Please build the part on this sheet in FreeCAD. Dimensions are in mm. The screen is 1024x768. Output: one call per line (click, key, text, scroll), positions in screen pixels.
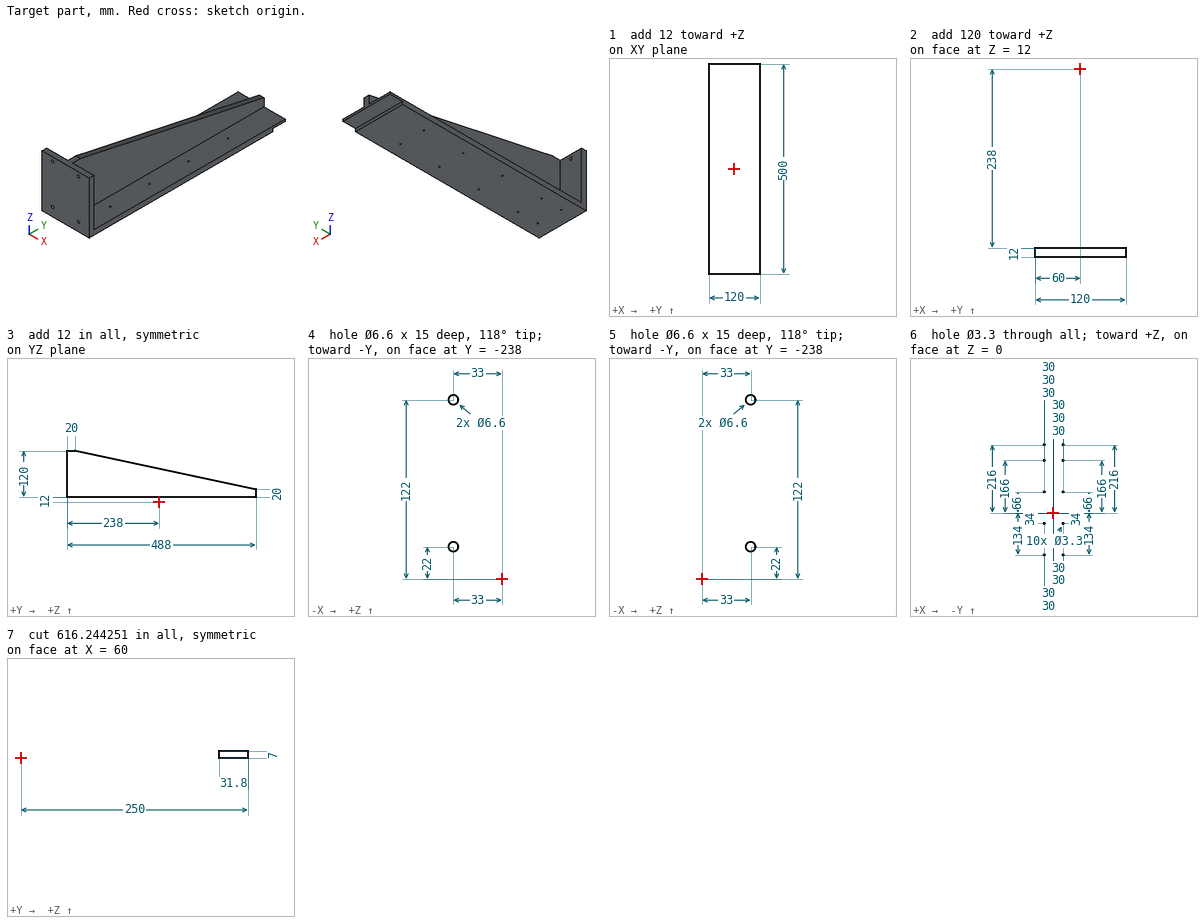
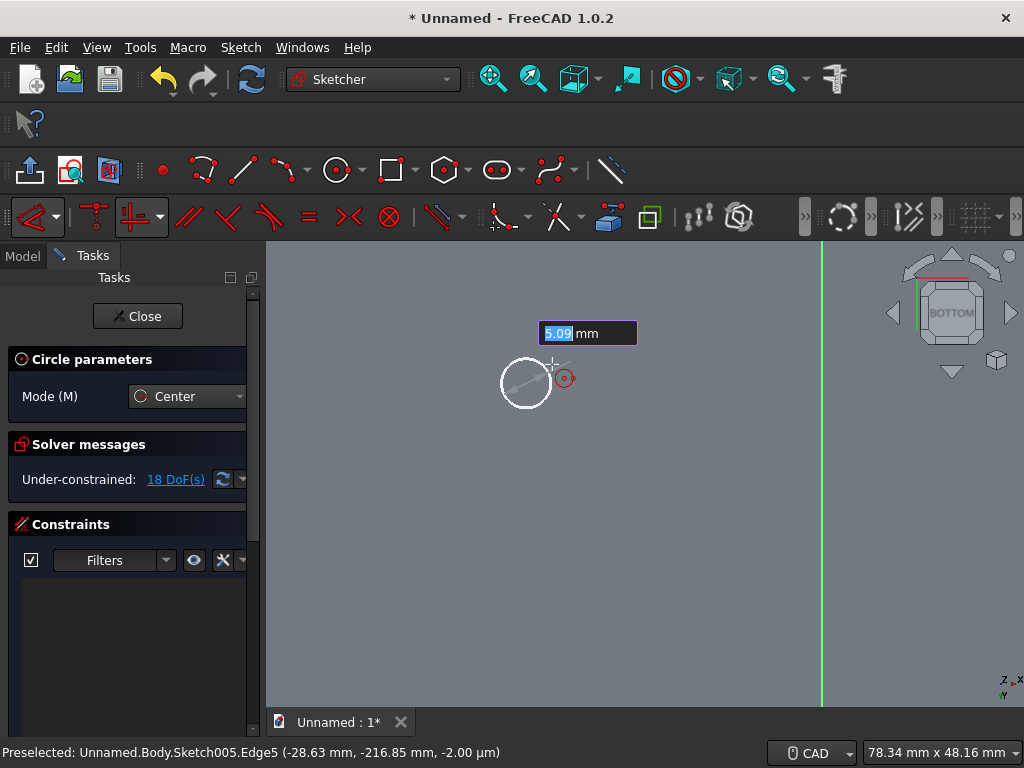
click(543, 356)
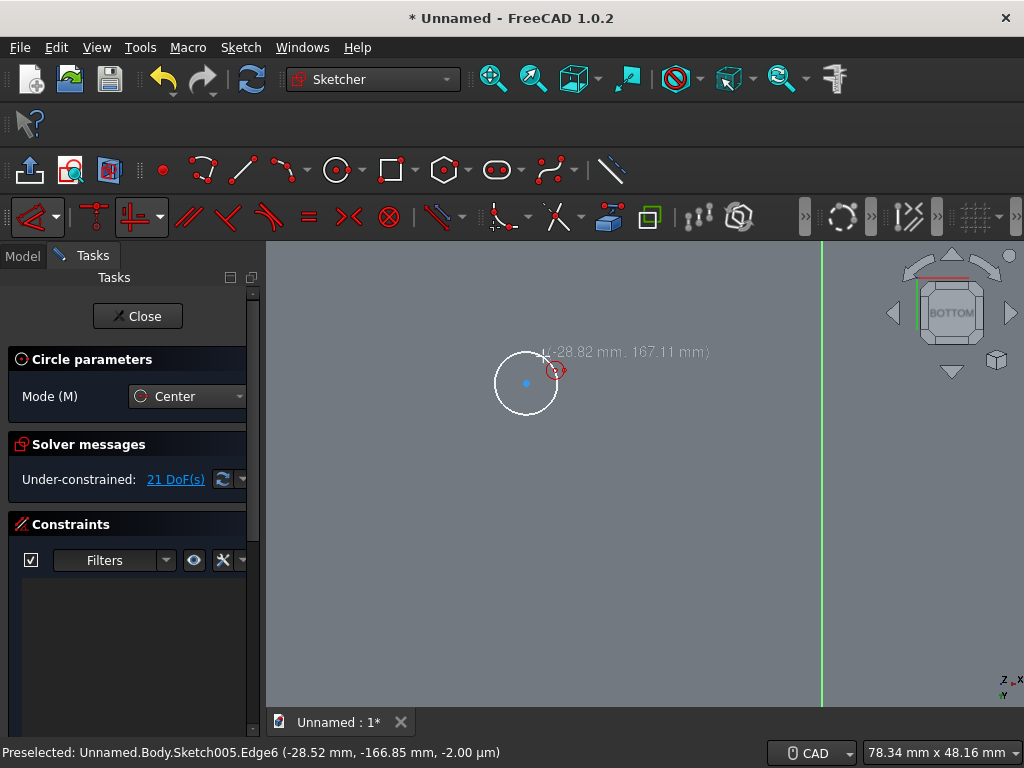
scroll(552, 364, down, 12)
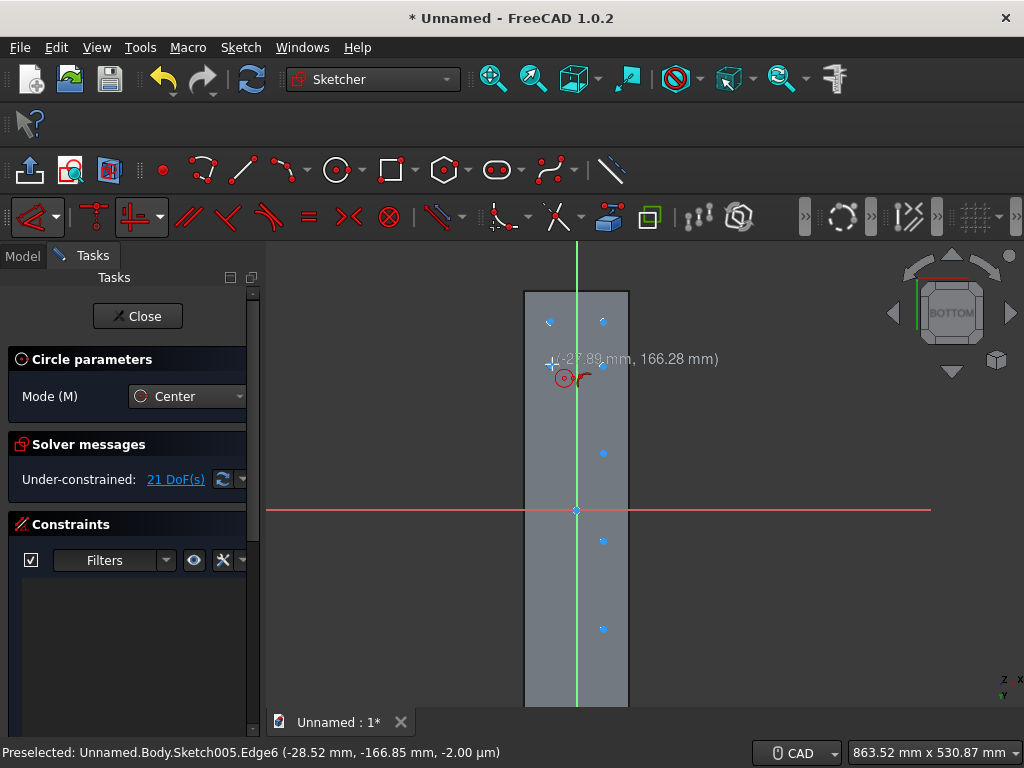
scroll(550, 452, up, 14)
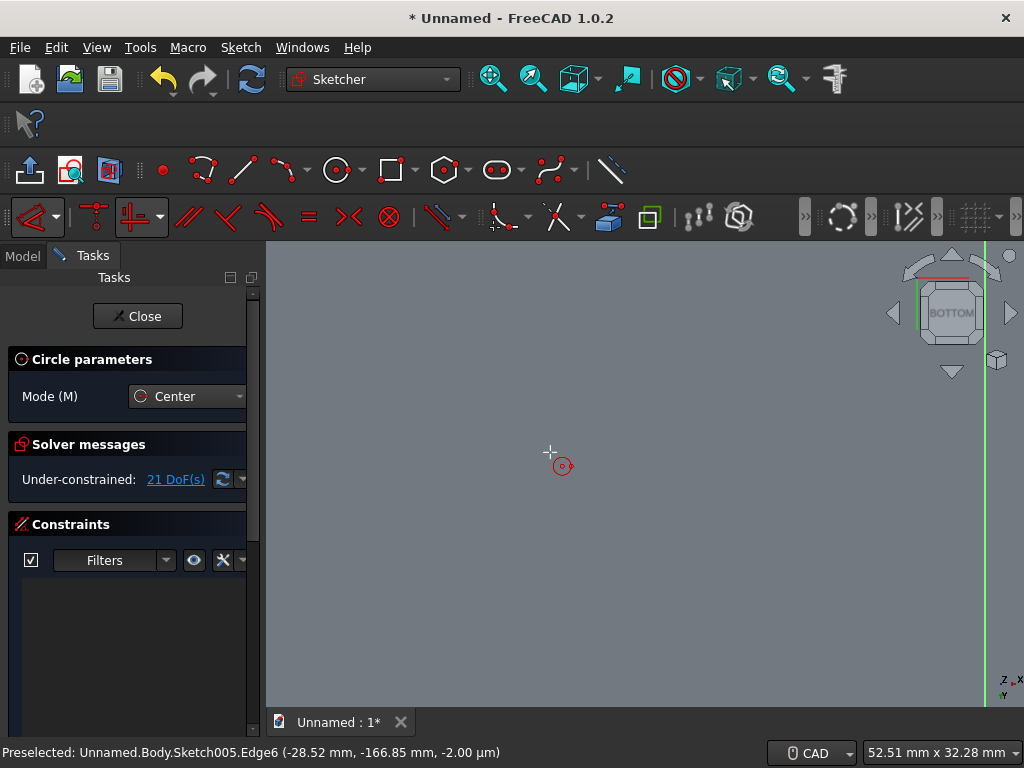
scroll(550, 452, down, 14)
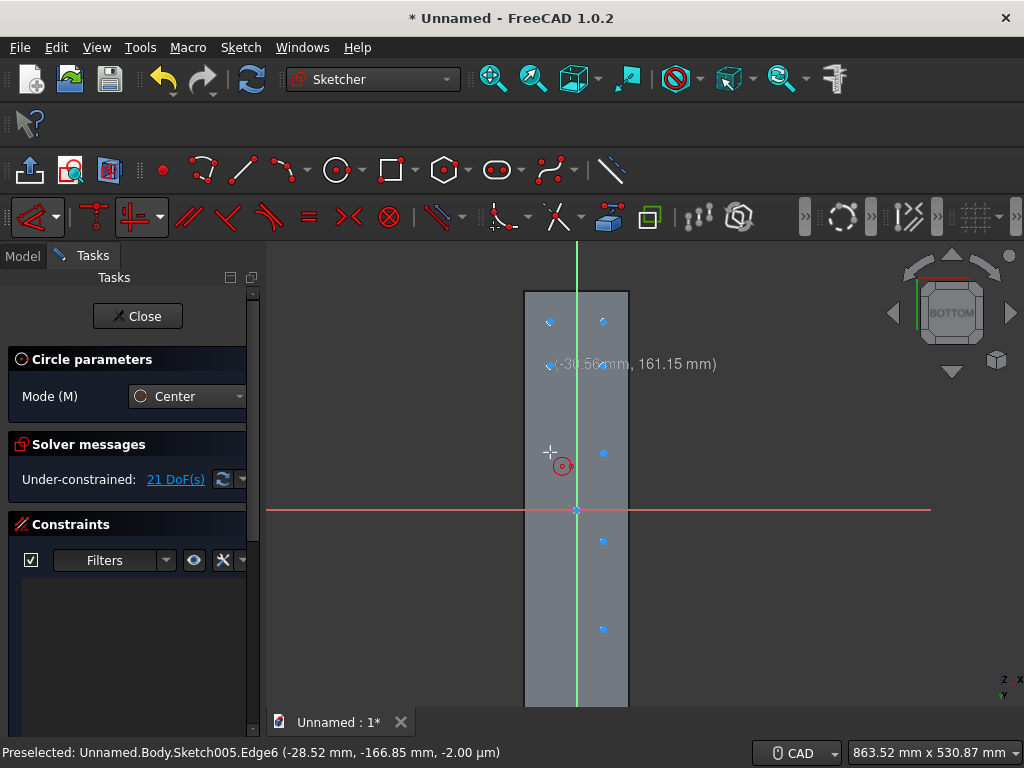
click(550, 452)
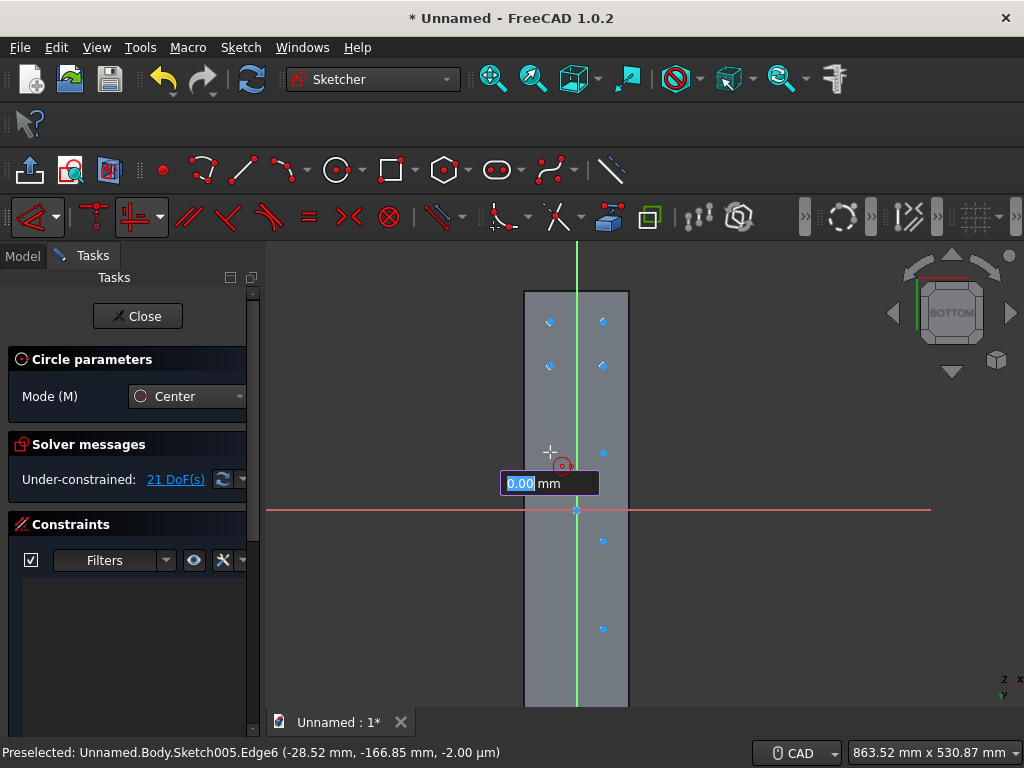
scroll(552, 451, up, 12)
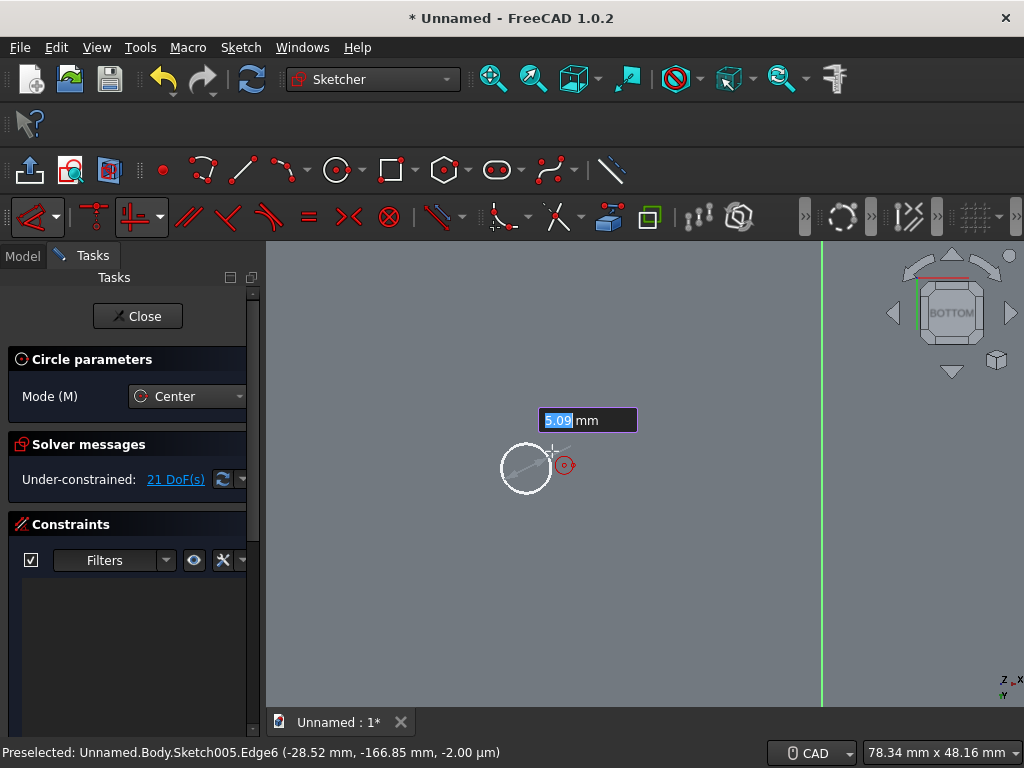
click(543, 450)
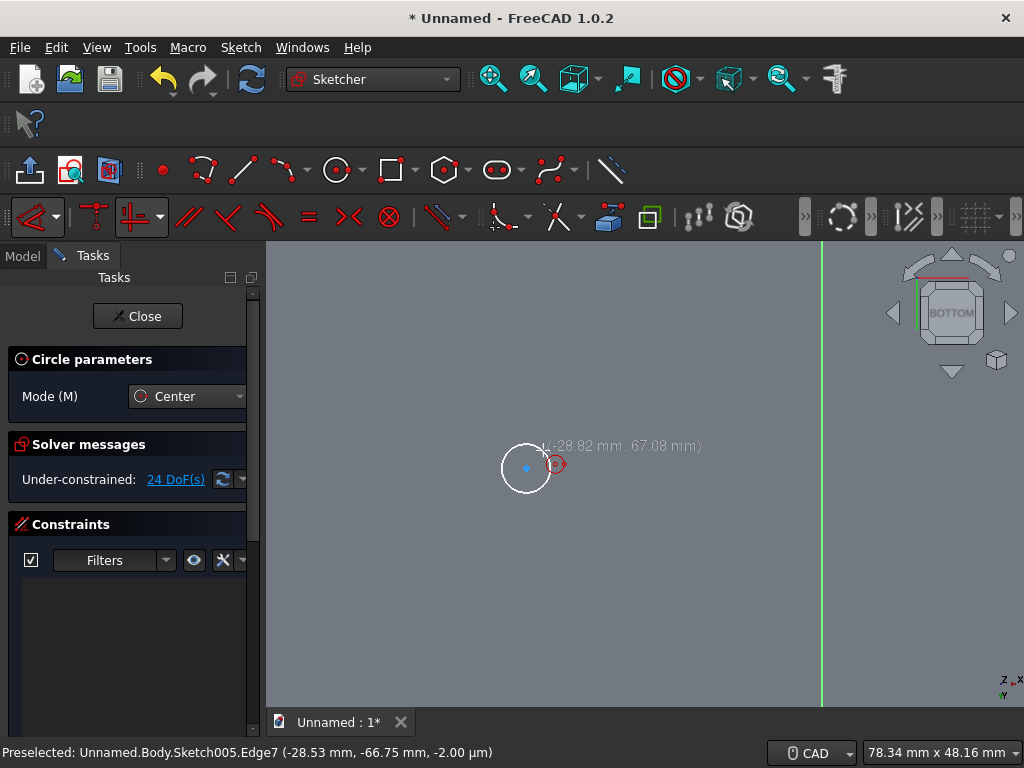
scroll(552, 451, down, 12)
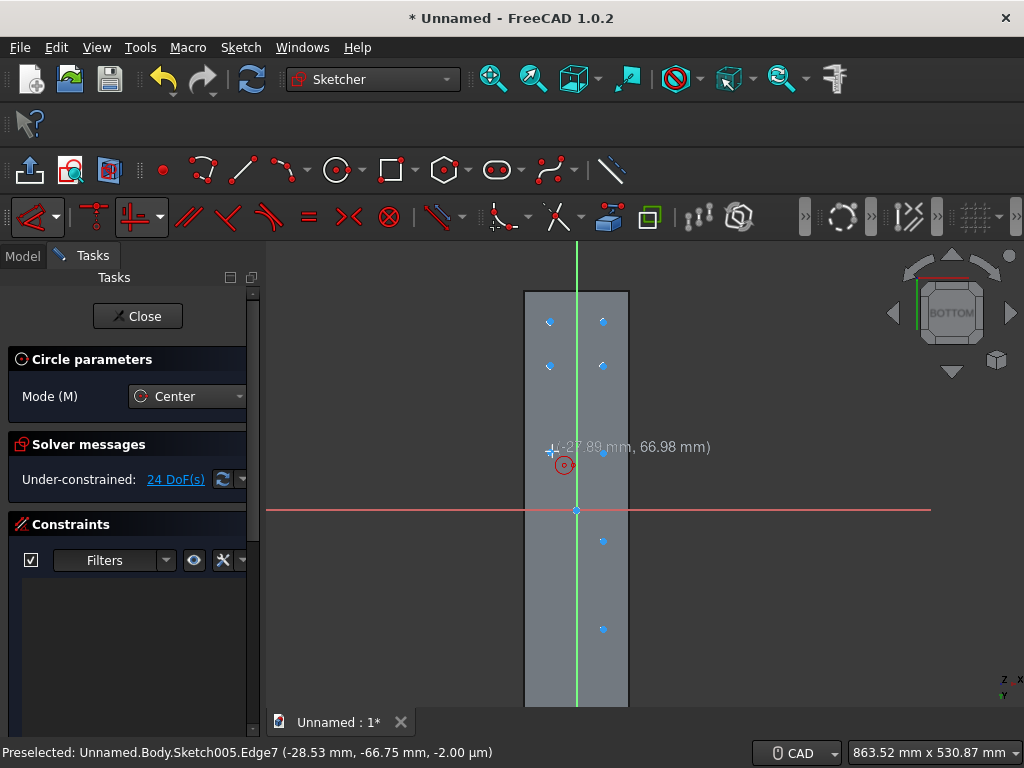
scroll(550, 540, up, 14)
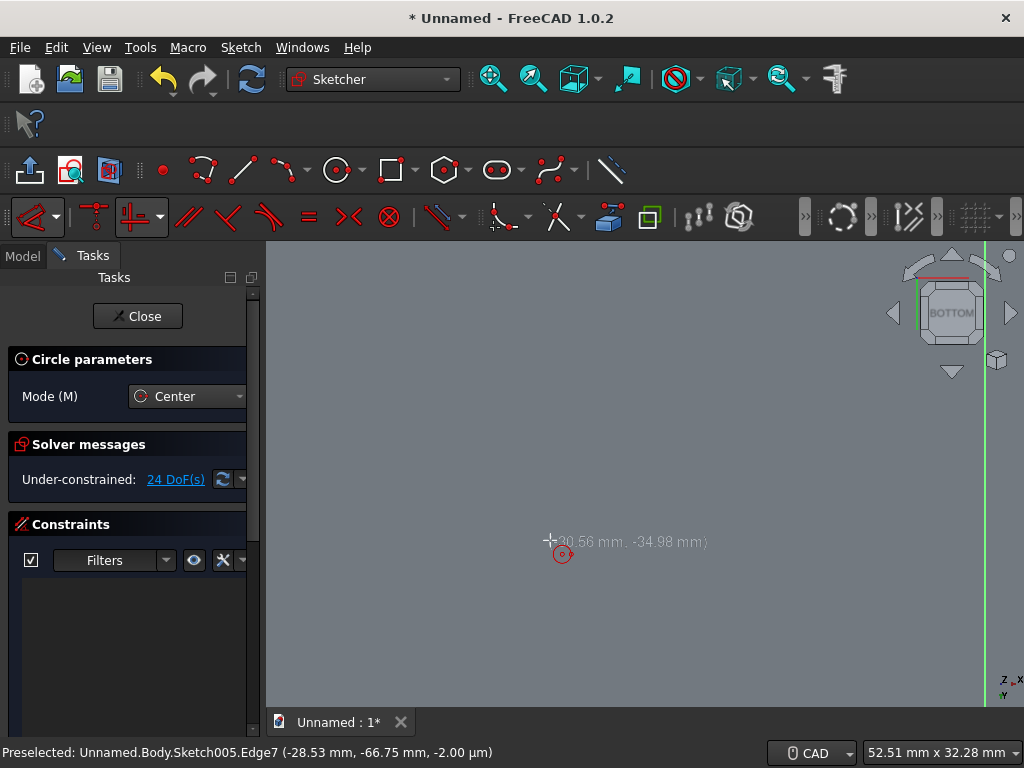
scroll(550, 540, down, 14)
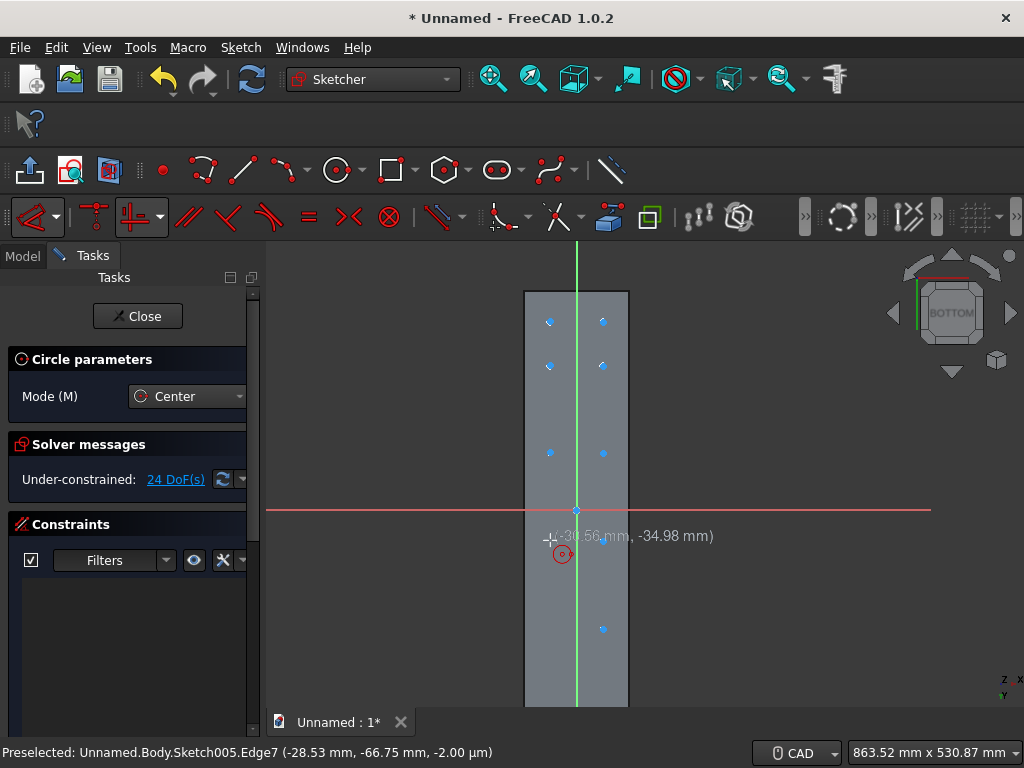
click(550, 540)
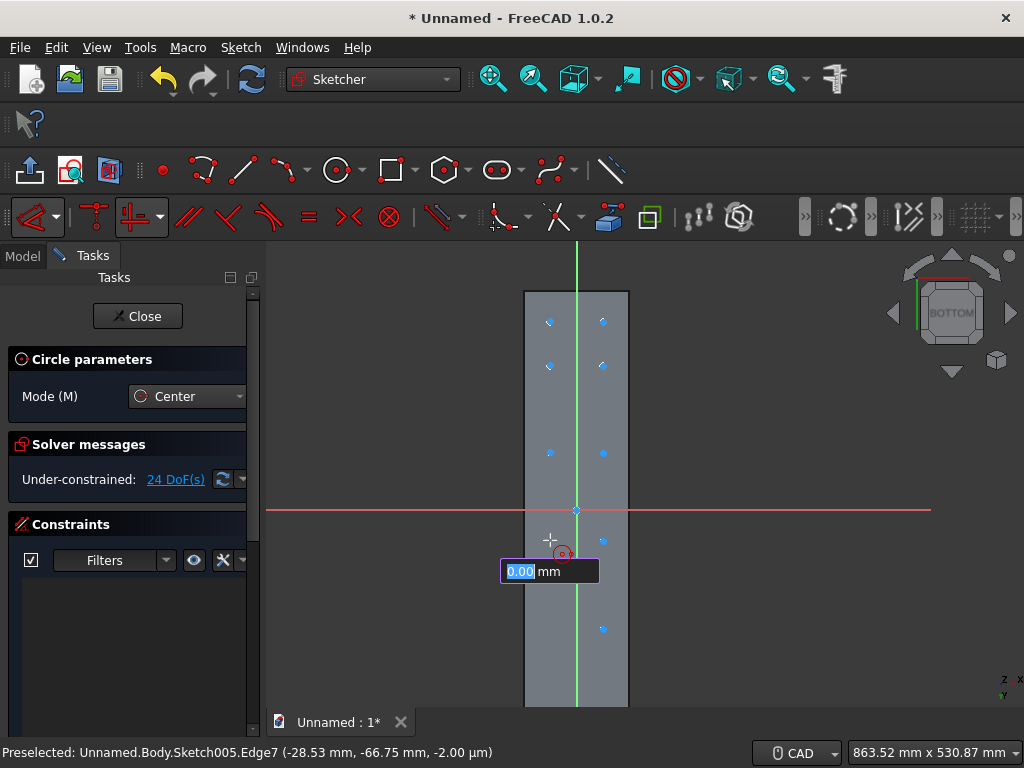
scroll(552, 539, up, 12)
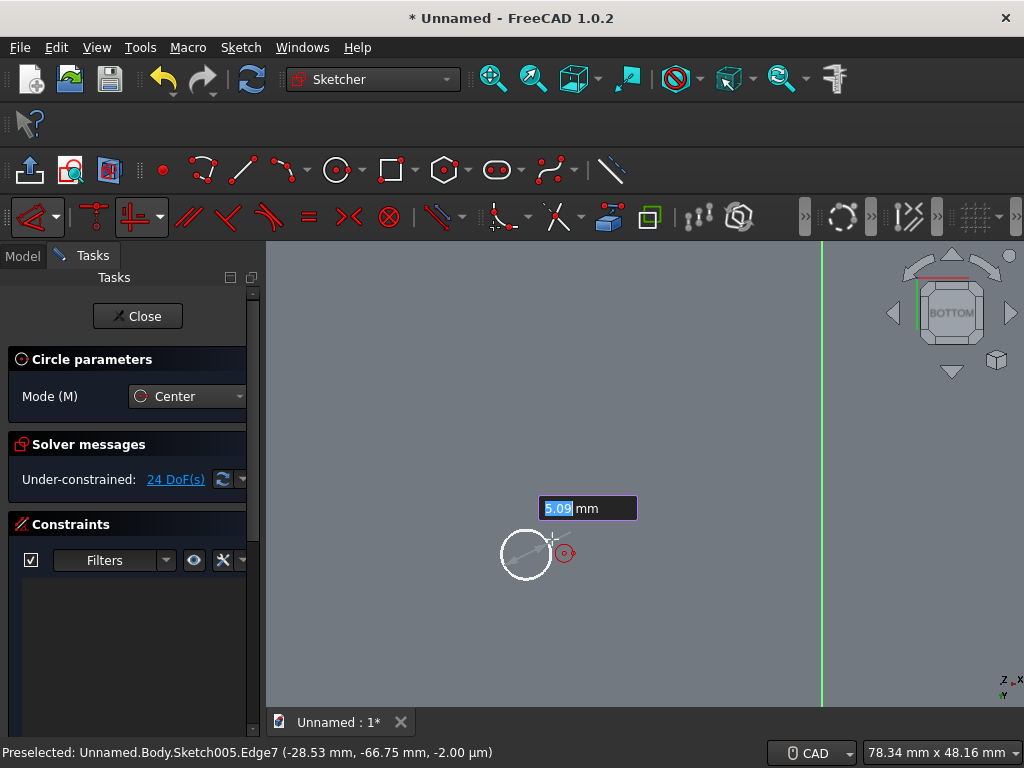
click(543, 534)